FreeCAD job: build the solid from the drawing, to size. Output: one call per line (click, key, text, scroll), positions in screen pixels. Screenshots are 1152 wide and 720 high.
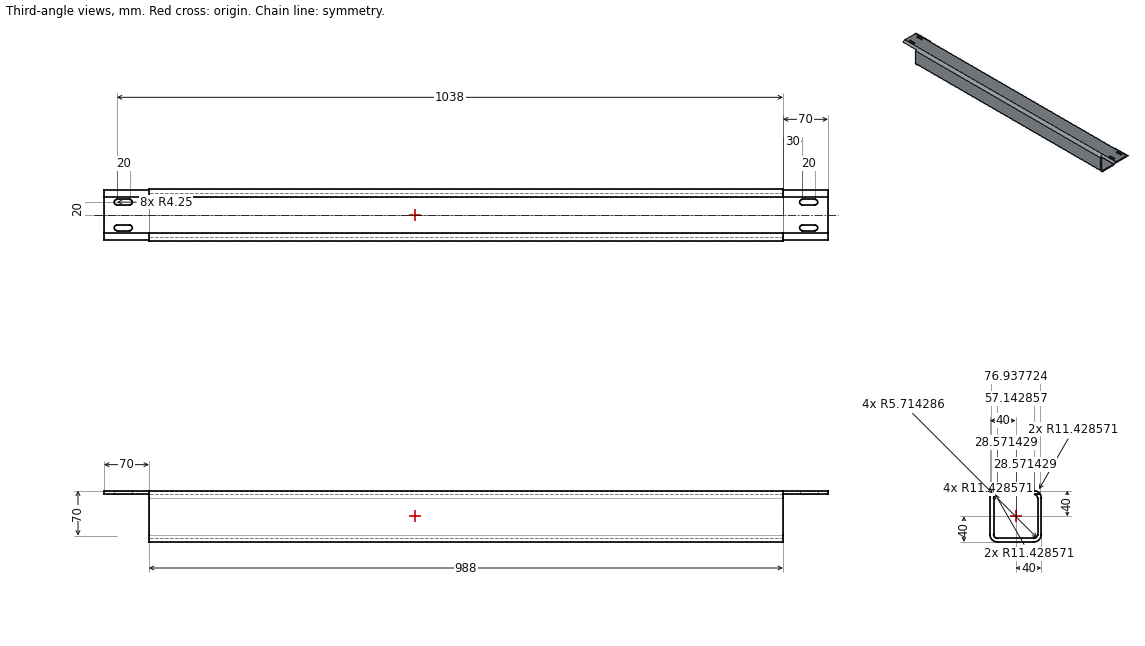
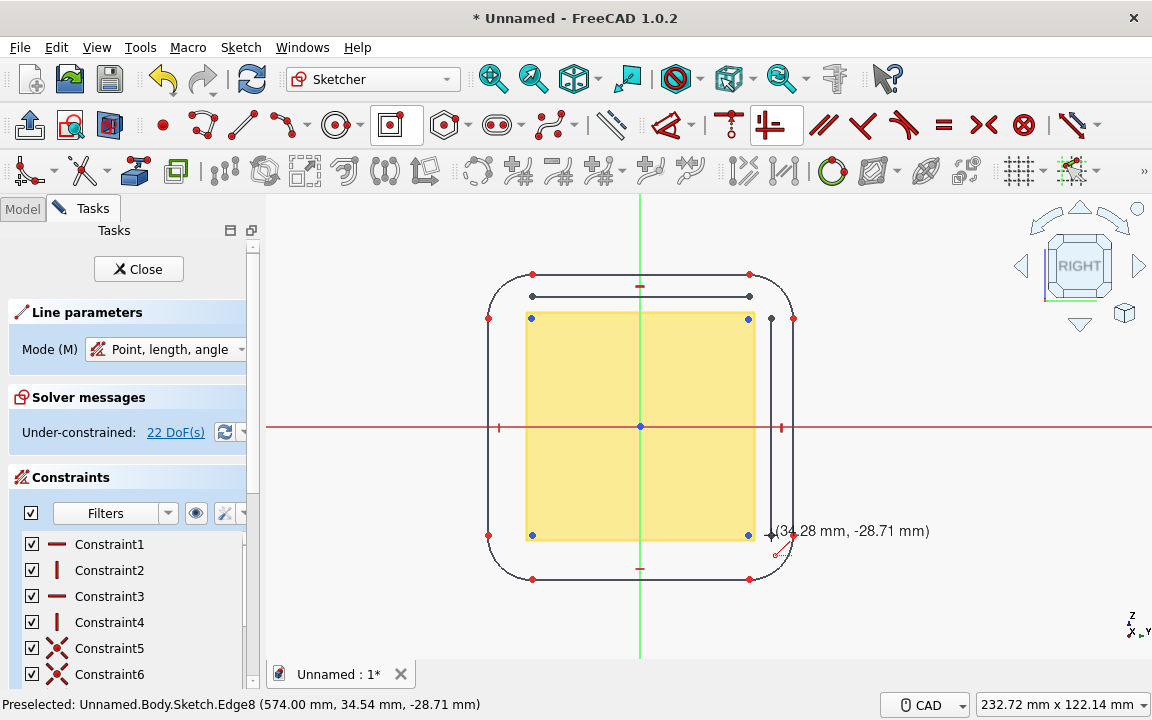
click(749, 557)
click(532, 557)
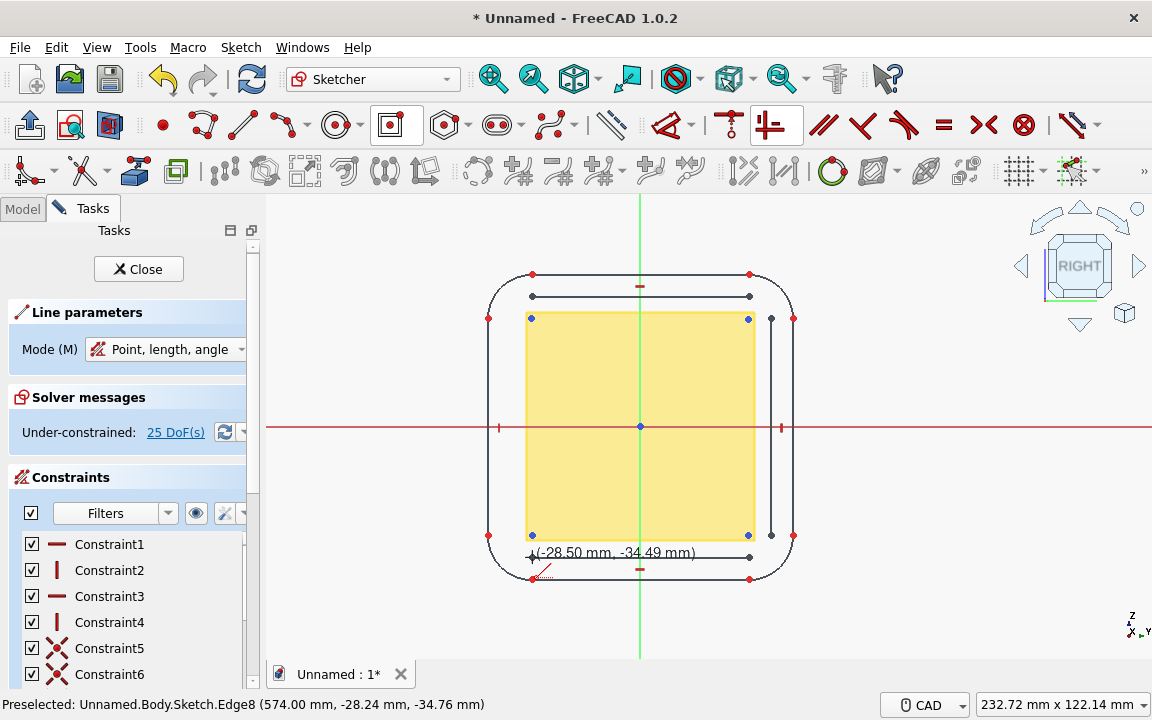
click(510, 535)
click(510, 318)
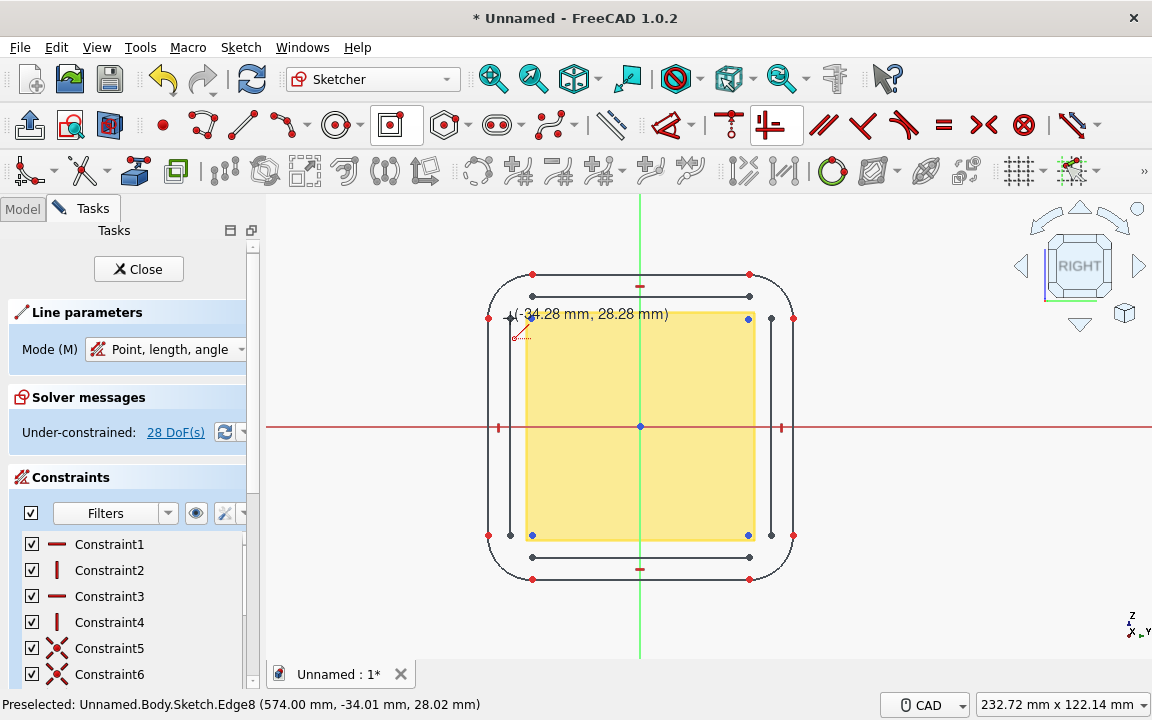
click(284, 126)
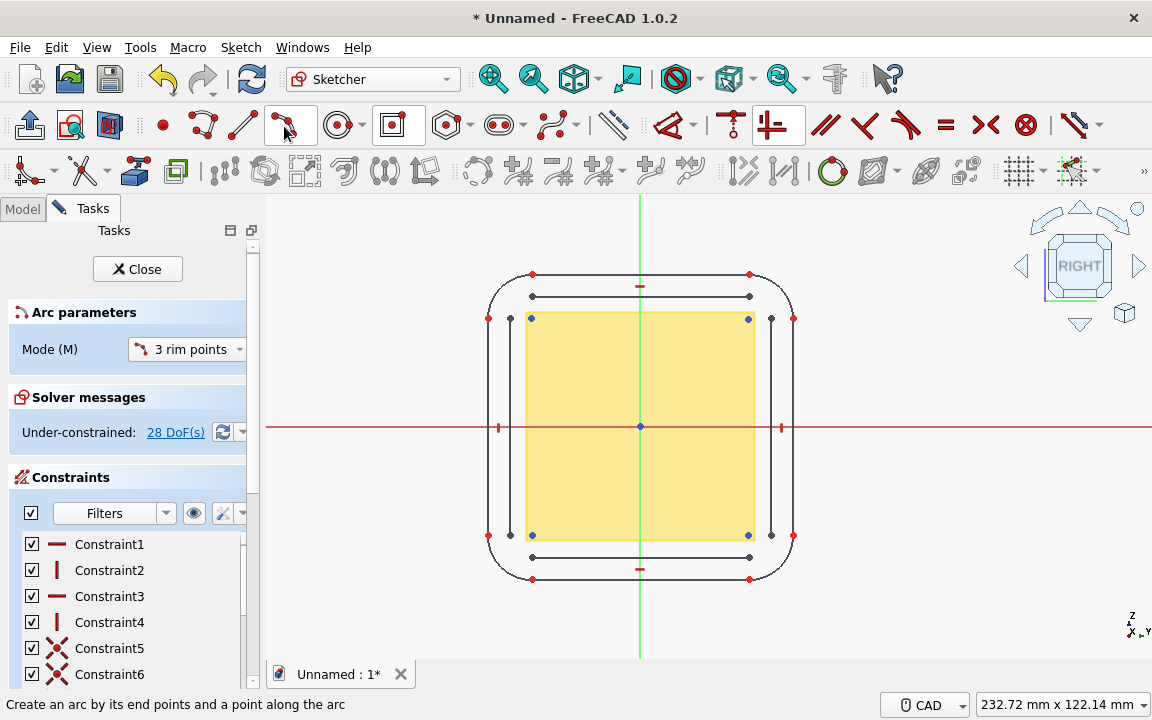
click(749, 297)
click(771, 319)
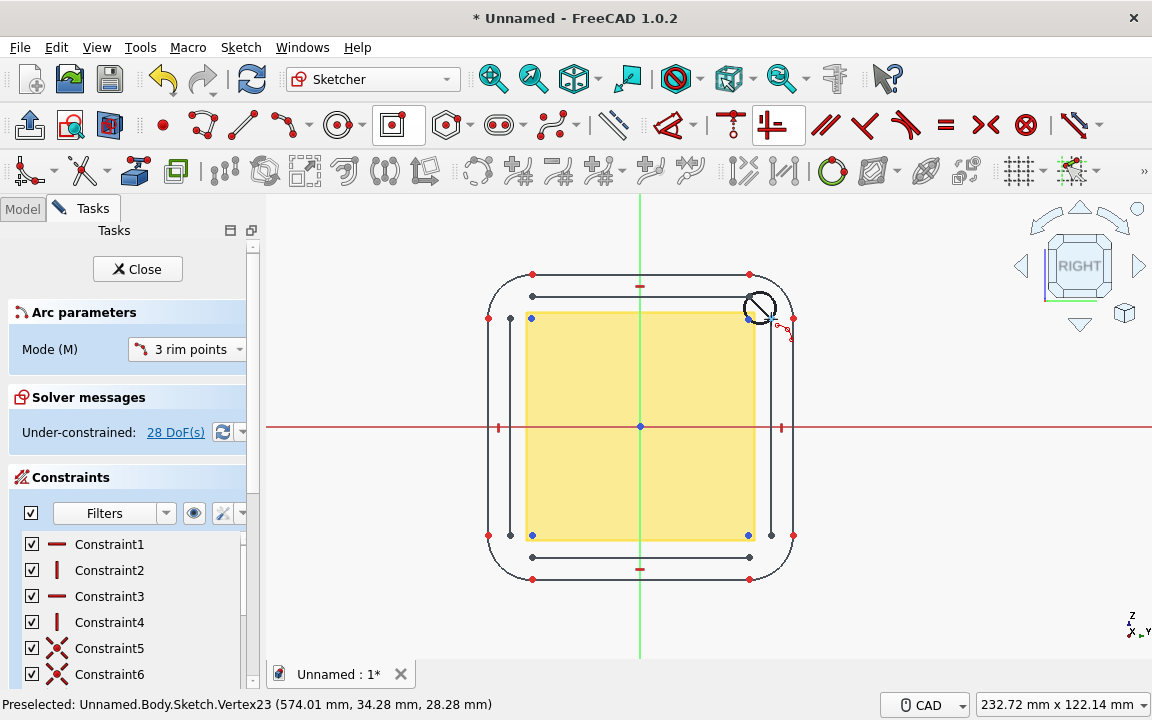
scroll(765, 303, up, 5)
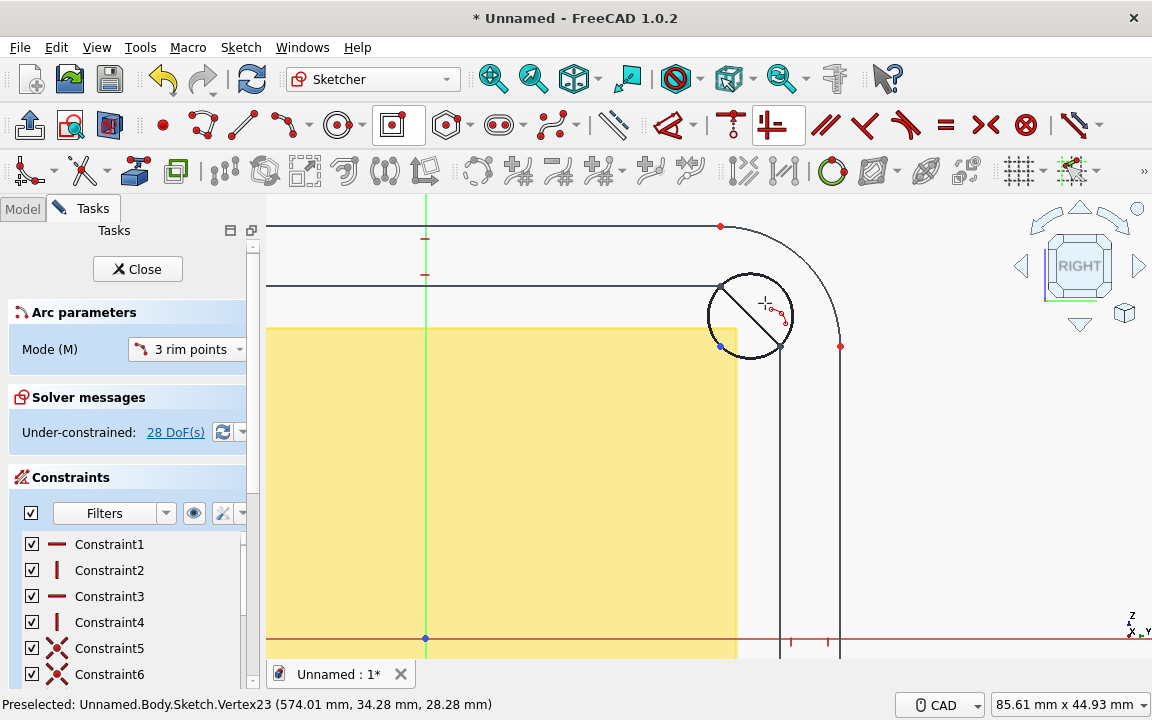
click(763, 301)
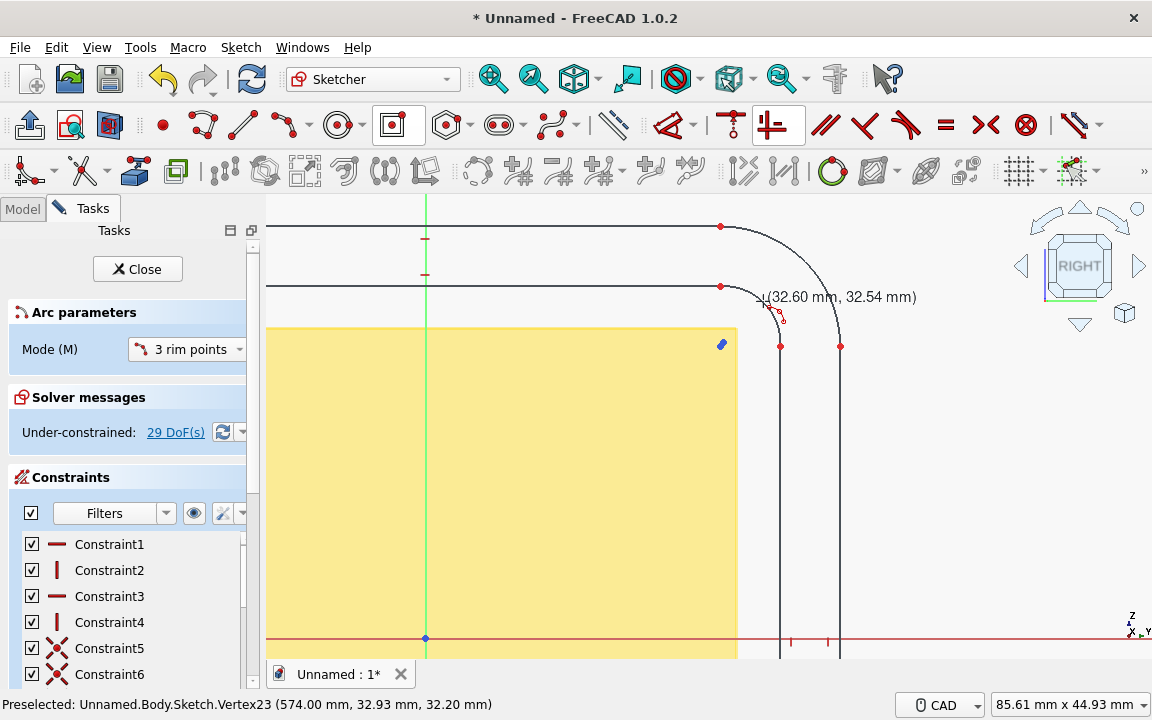
scroll(766, 303, down, 5)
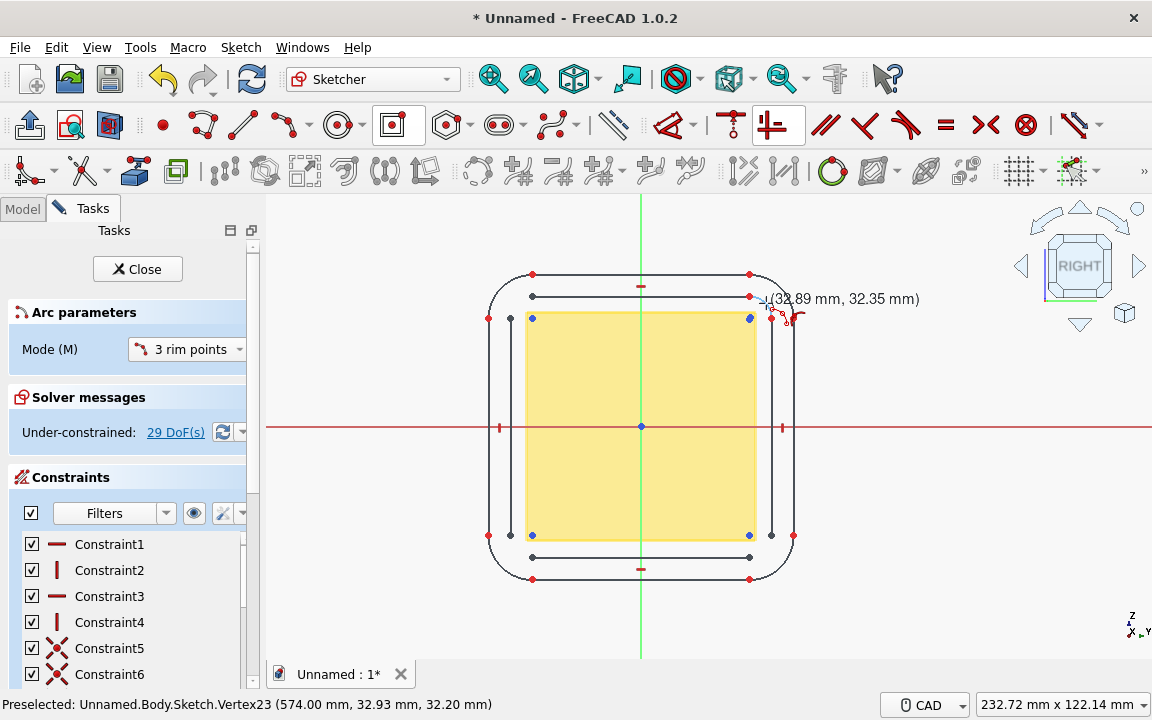
click(772, 536)
click(750, 558)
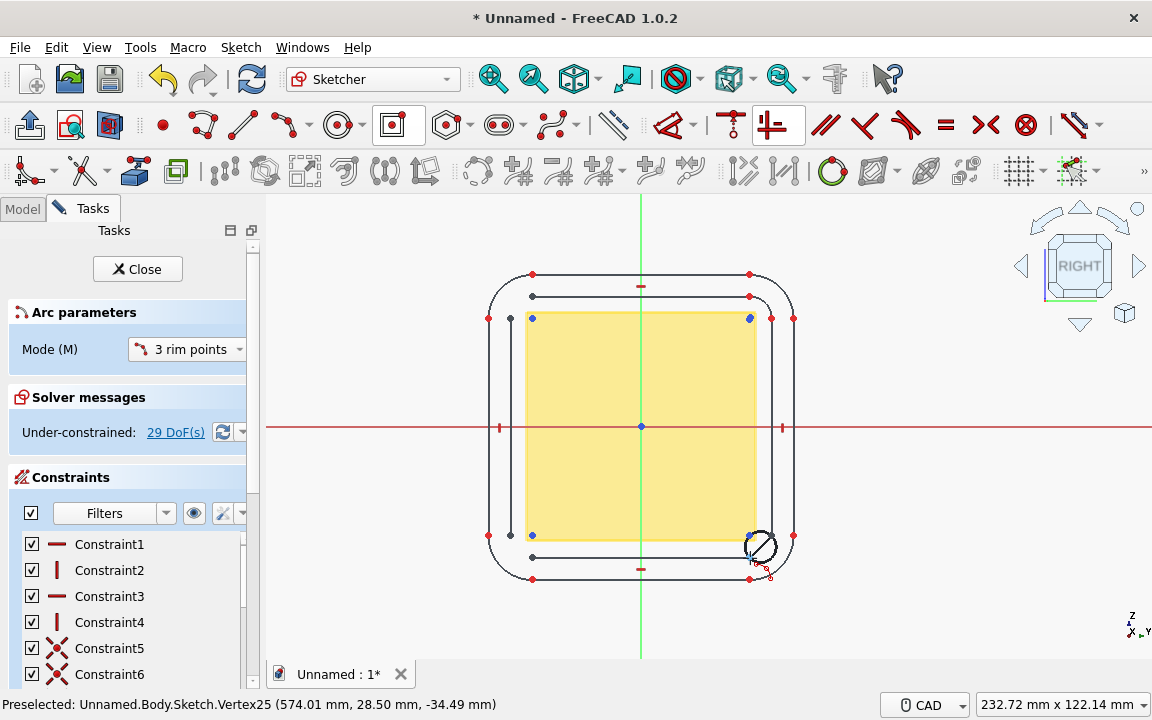
scroll(765, 551, up, 5)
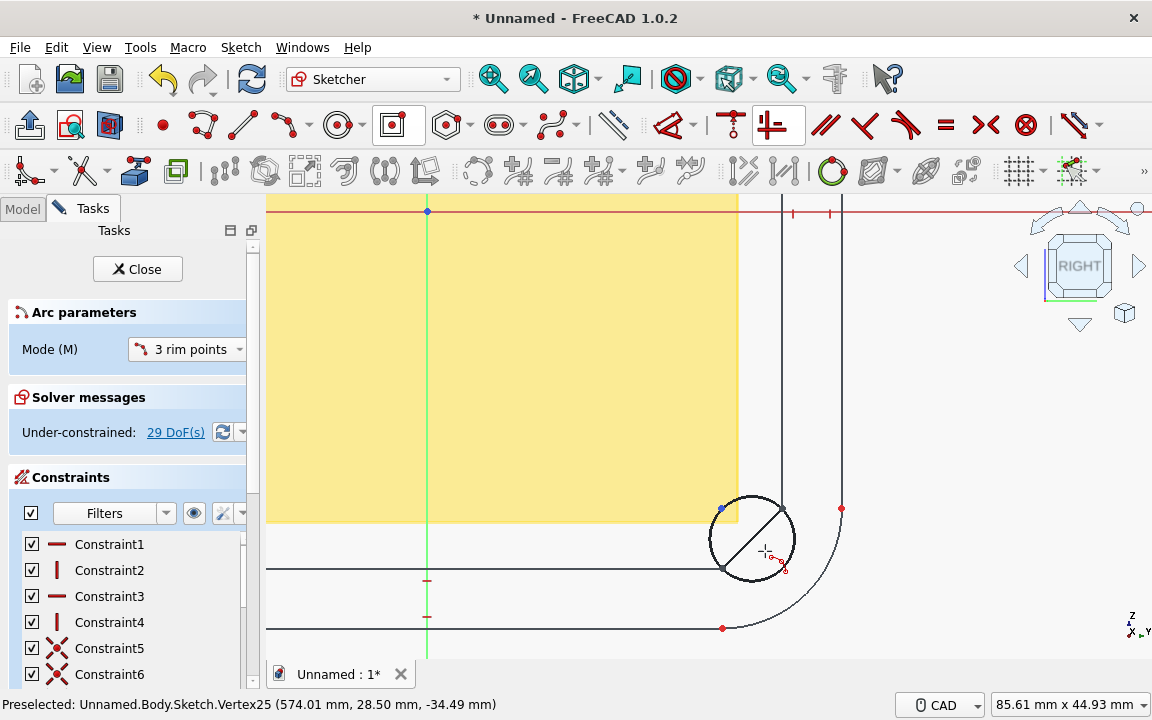
click(765, 549)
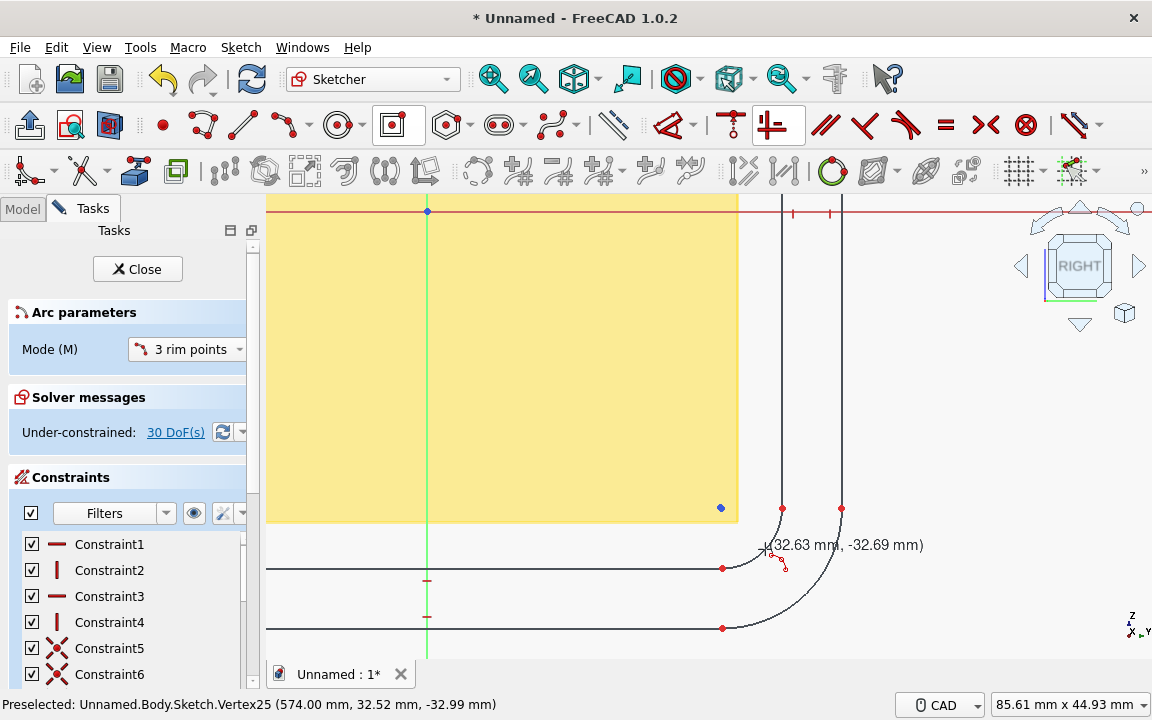
scroll(765, 551, down, 5)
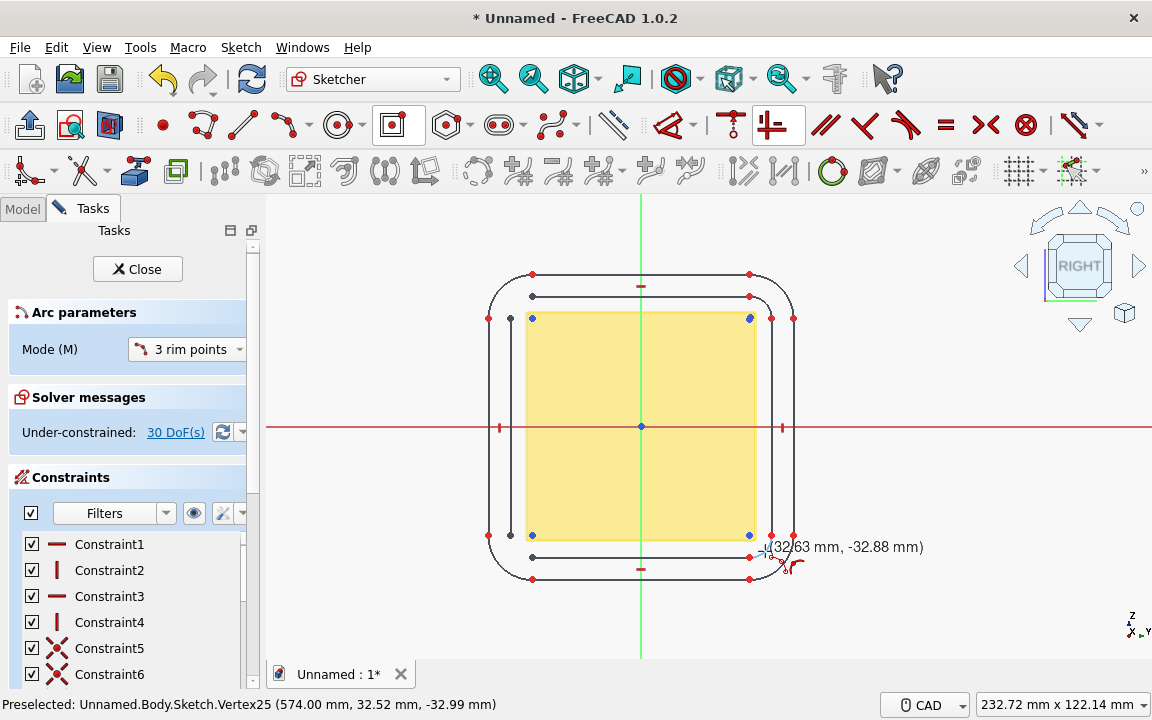
click(533, 558)
click(511, 536)